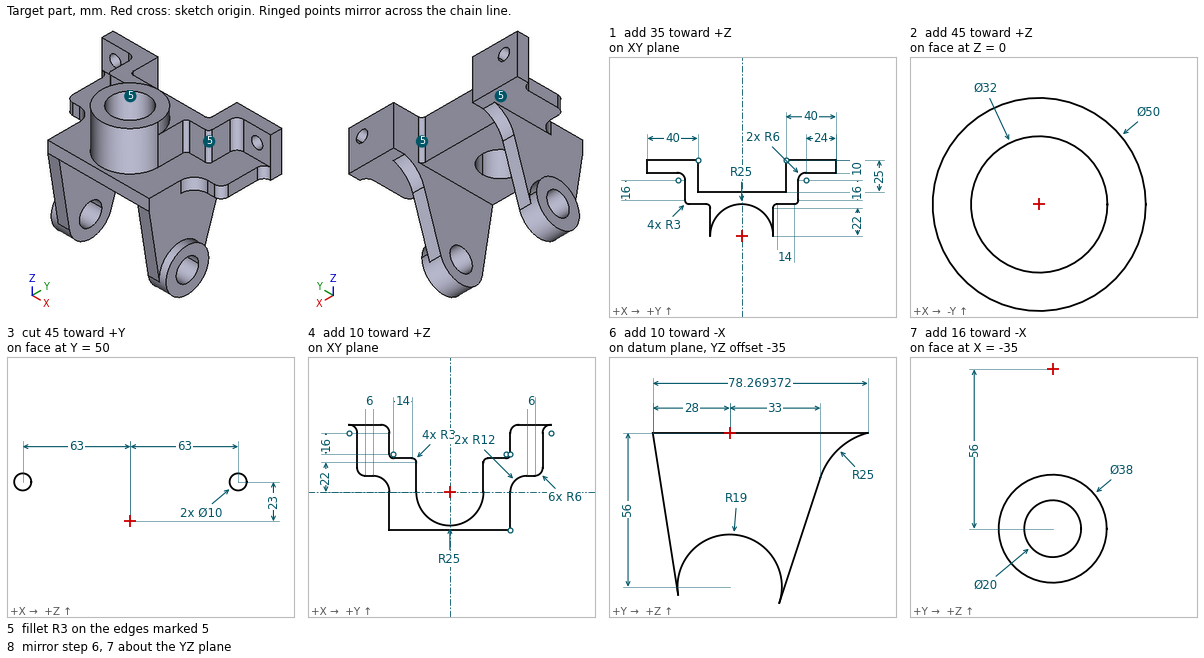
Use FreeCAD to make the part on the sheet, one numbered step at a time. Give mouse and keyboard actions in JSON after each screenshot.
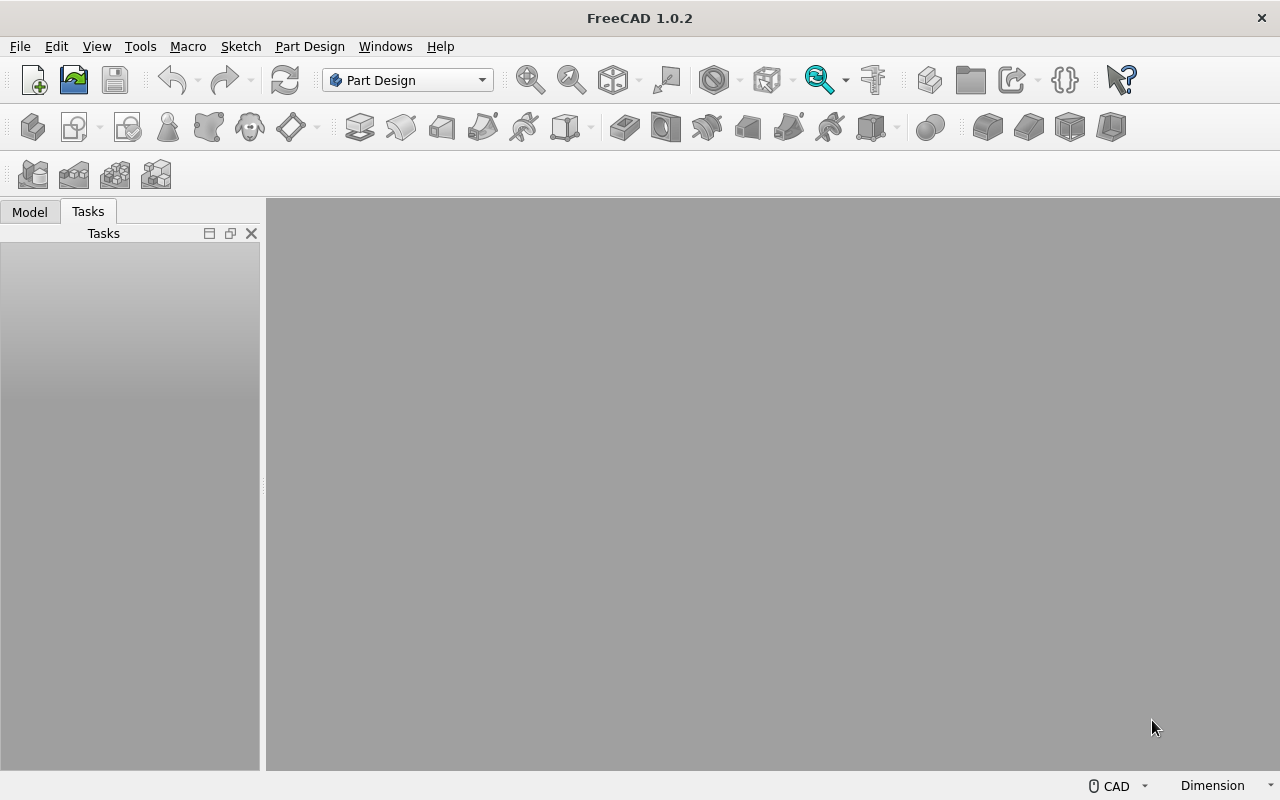
{"action": "left_click", "coordinate": [33, 80]}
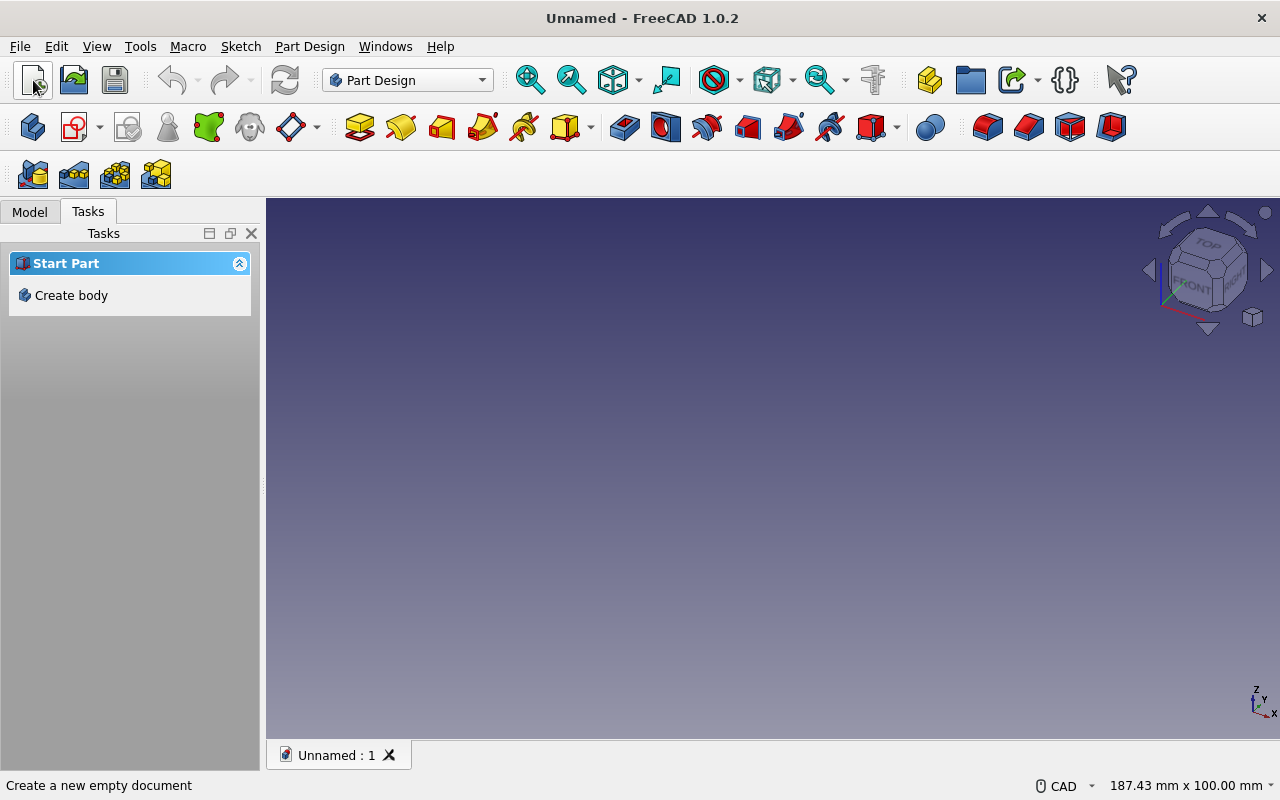
{"action": "left_click", "coordinate": [74, 128]}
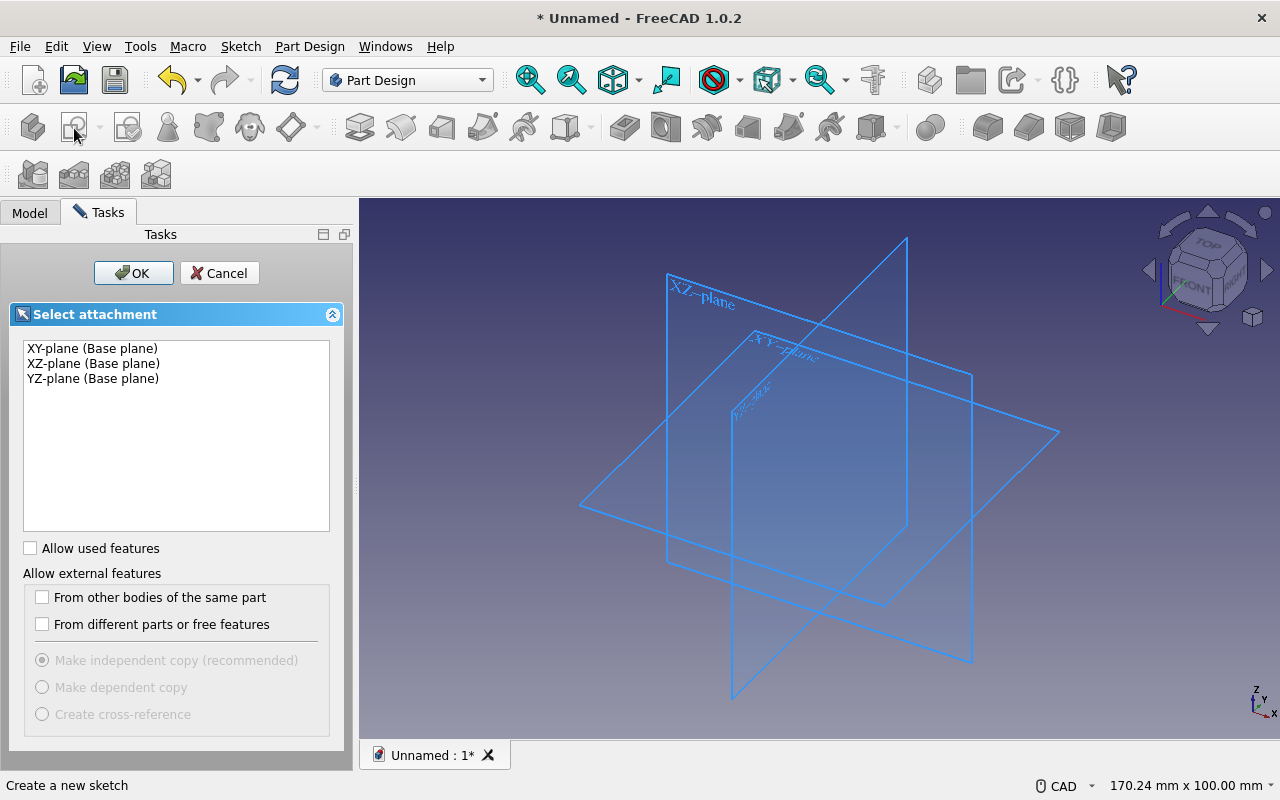
{"action": "left_click", "coordinate": [84, 348]}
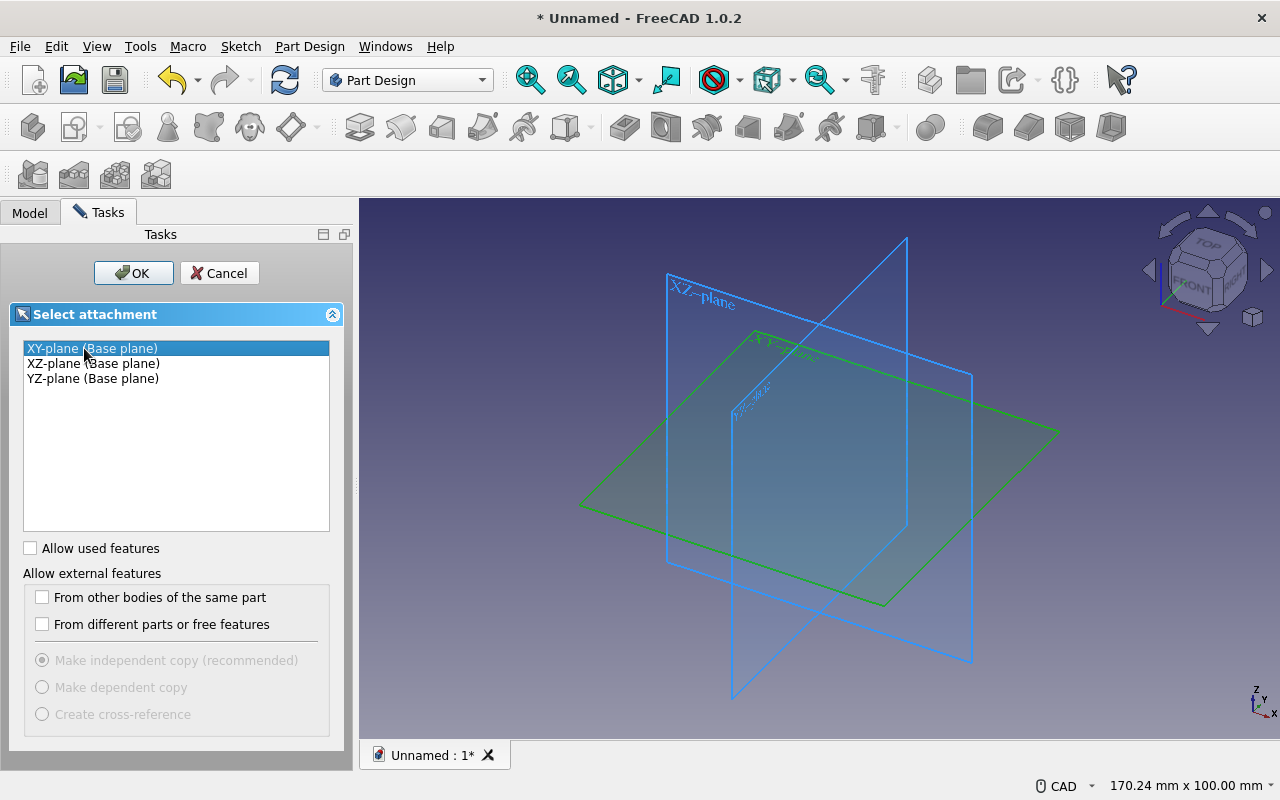
{"action": "left_click", "coordinate": [134, 273]}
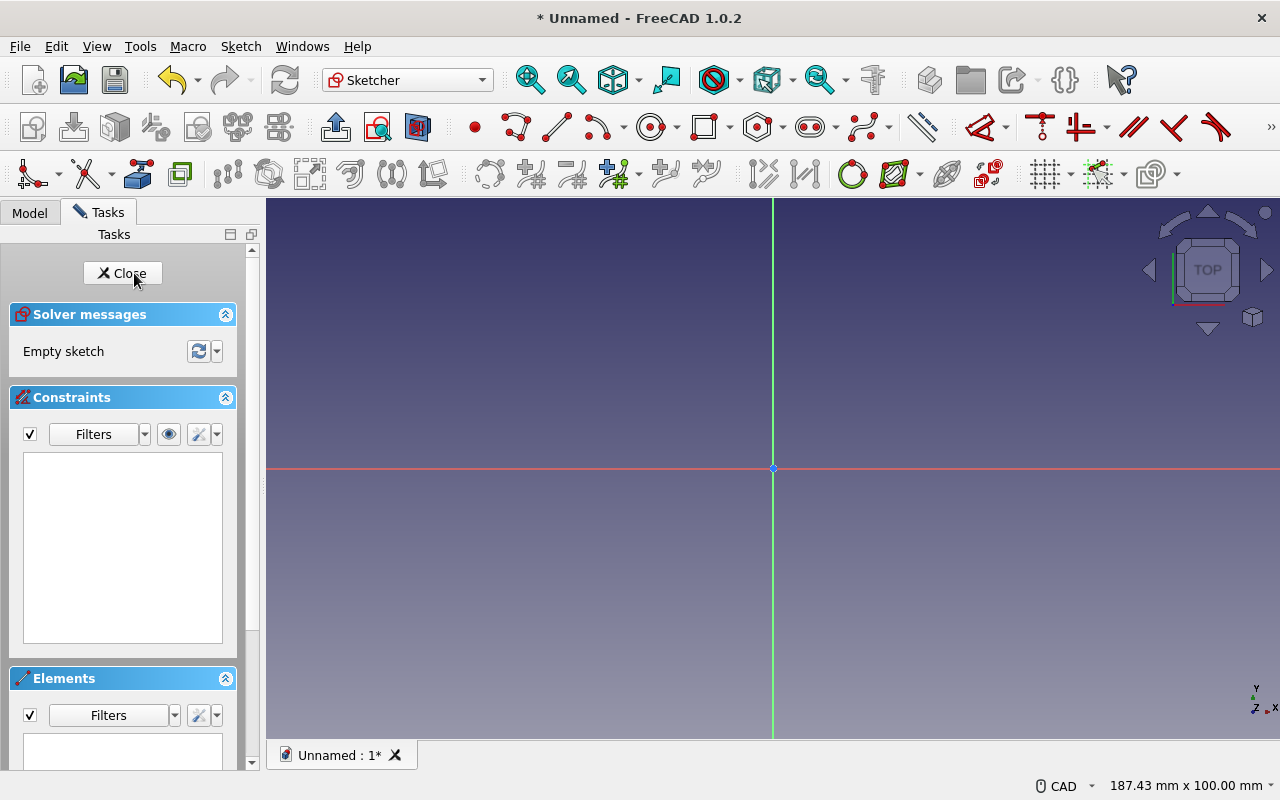
{"action": "scroll", "coordinate": [565, 711], "scroll_direction": "down", "scroll_amount": 2}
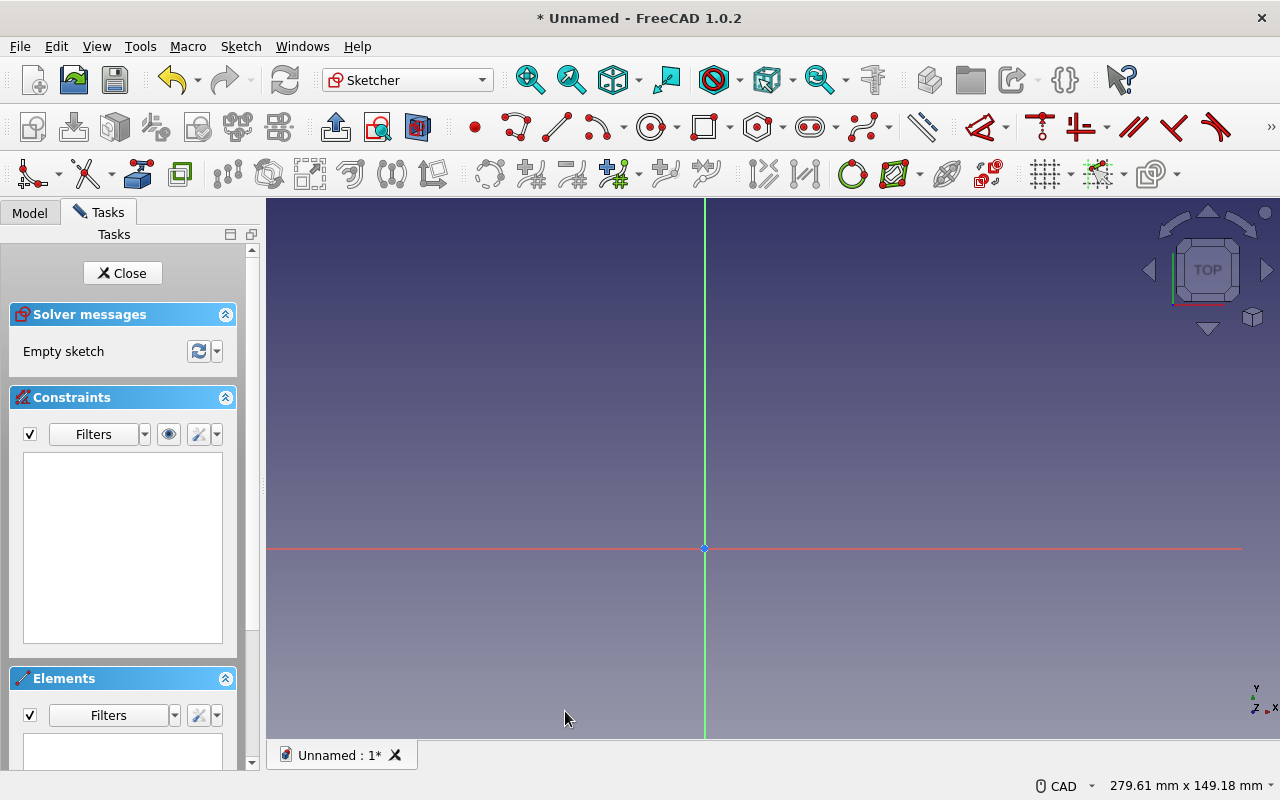
{"action": "left_click", "coordinate": [557, 128]}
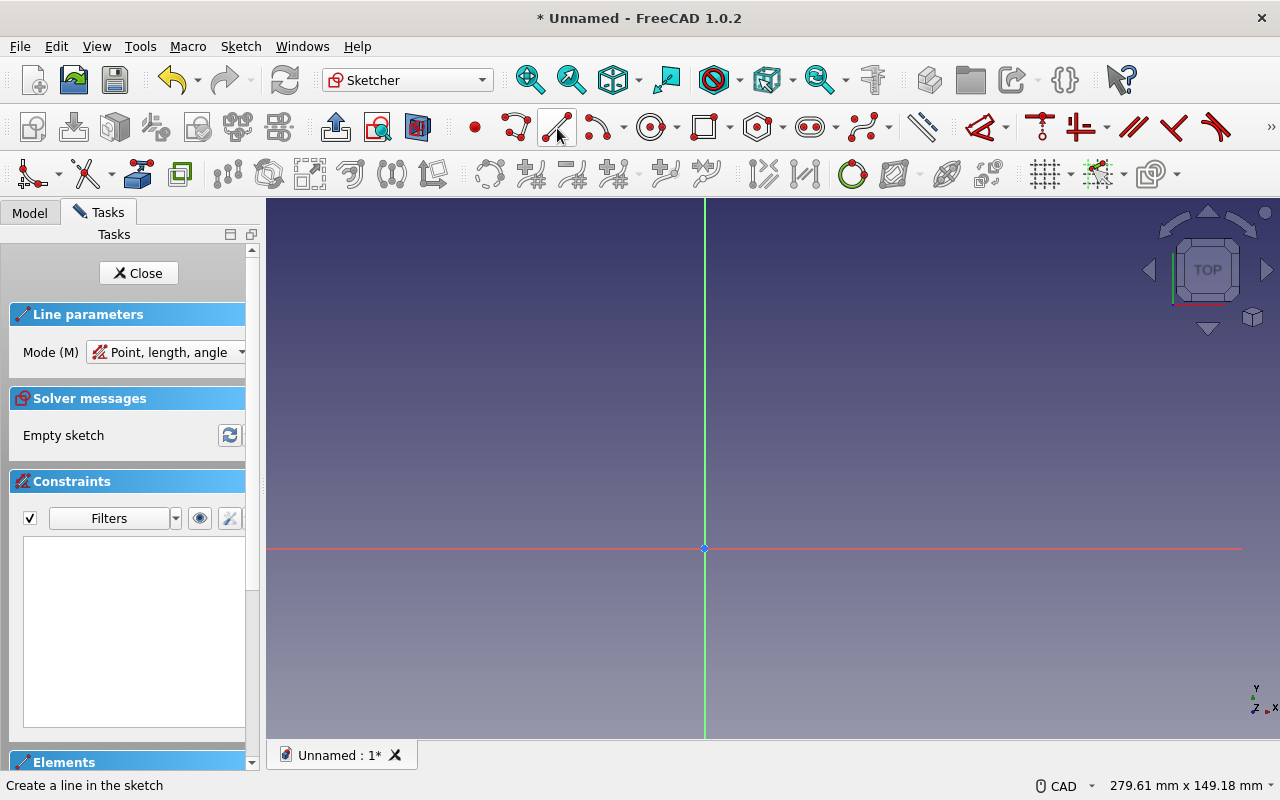
{"action": "left_click", "coordinate": [795, 549]}
{"action": "left_click", "coordinate": [795, 469]}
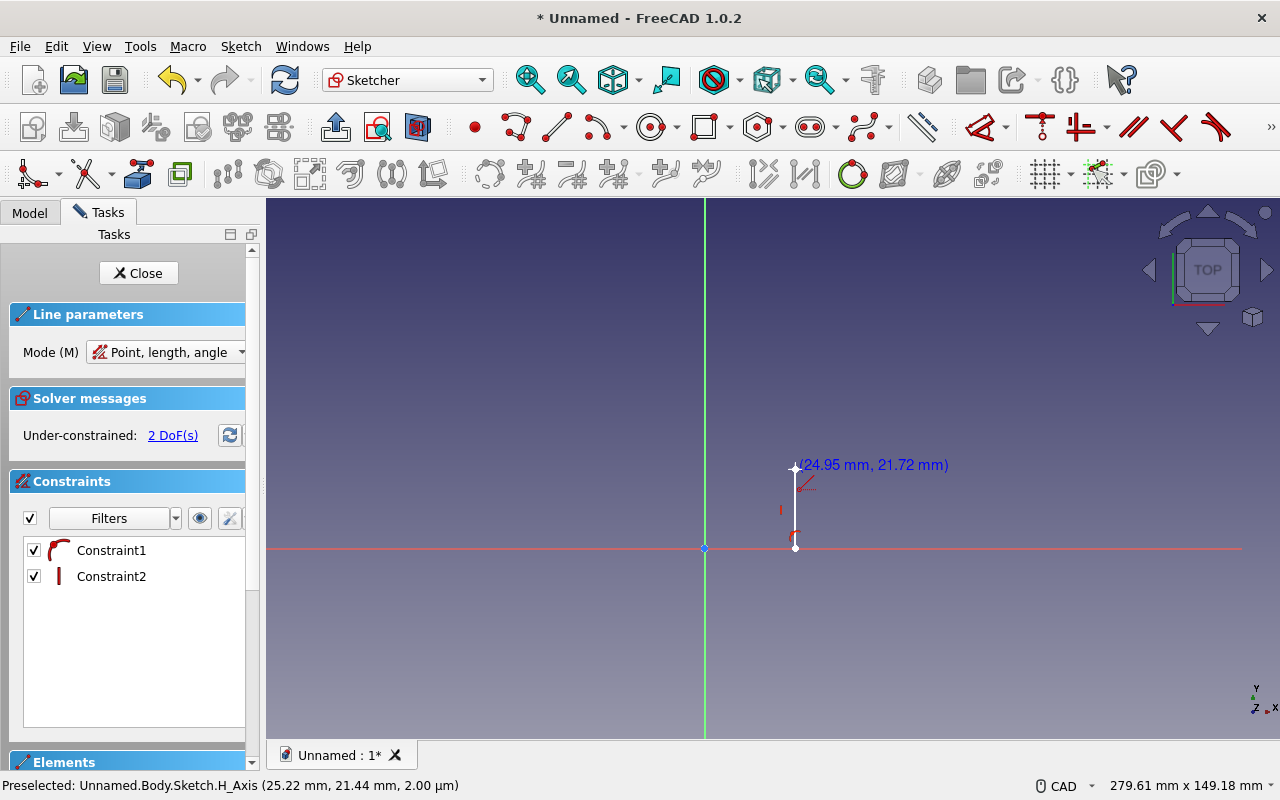
{"action": "left_click", "coordinate": [806, 458]}
{"action": "left_click", "coordinate": [857, 458]}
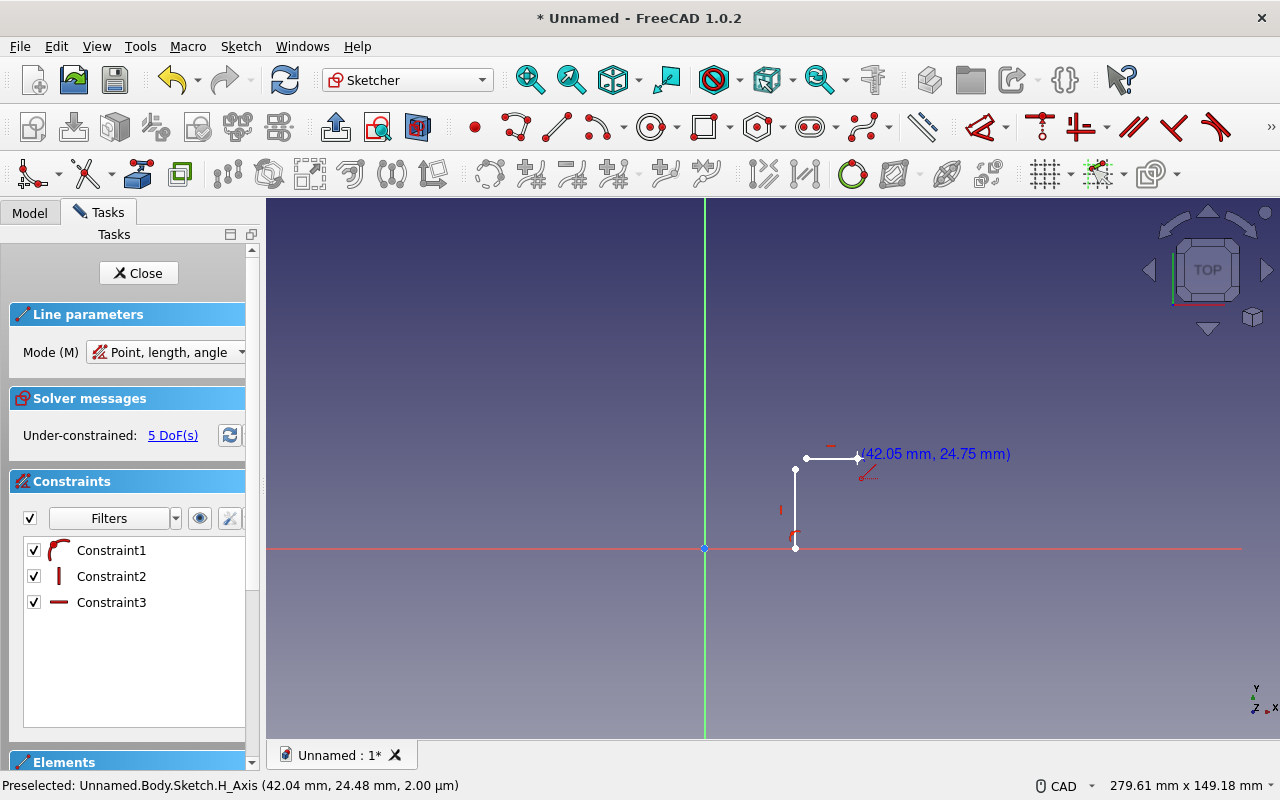
{"action": "left_click", "coordinate": [868, 447]}
{"action": "left_click", "coordinate": [868, 389]}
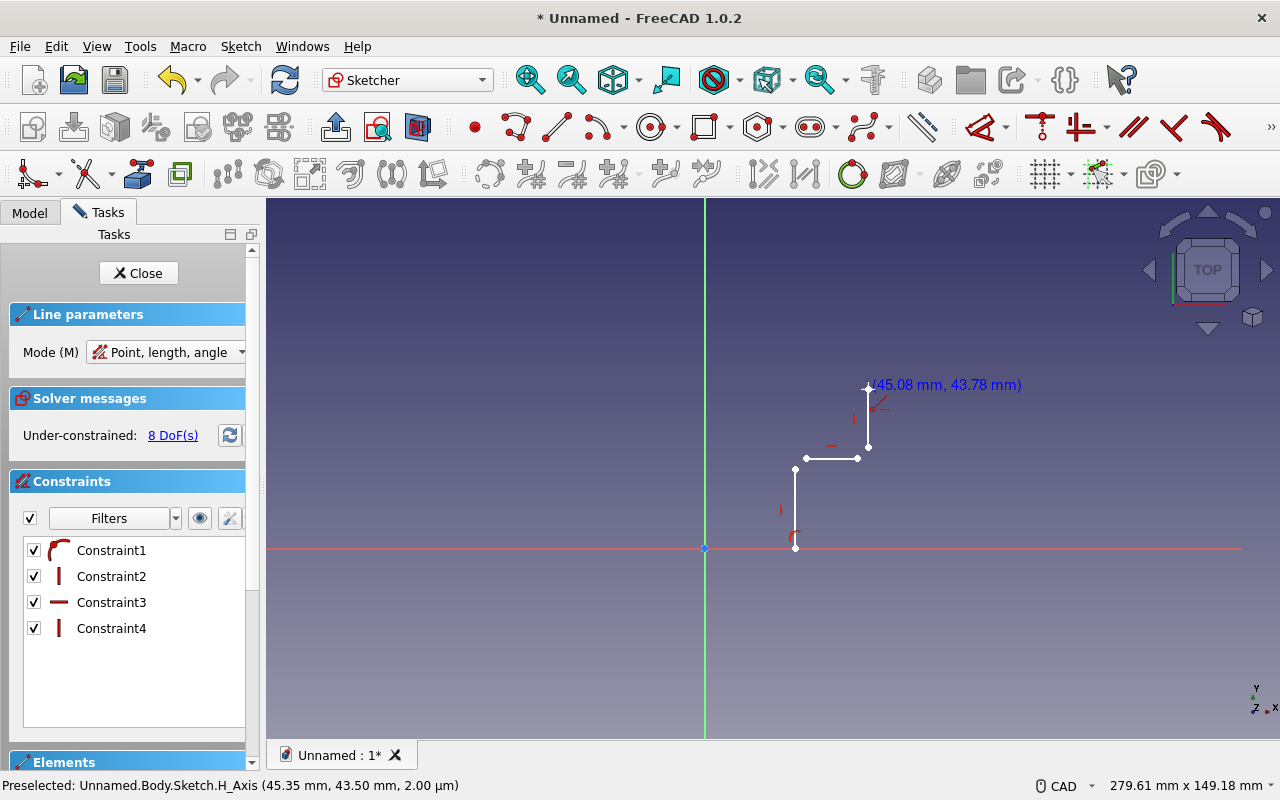
{"action": "left_click", "coordinate": [516, 128]}